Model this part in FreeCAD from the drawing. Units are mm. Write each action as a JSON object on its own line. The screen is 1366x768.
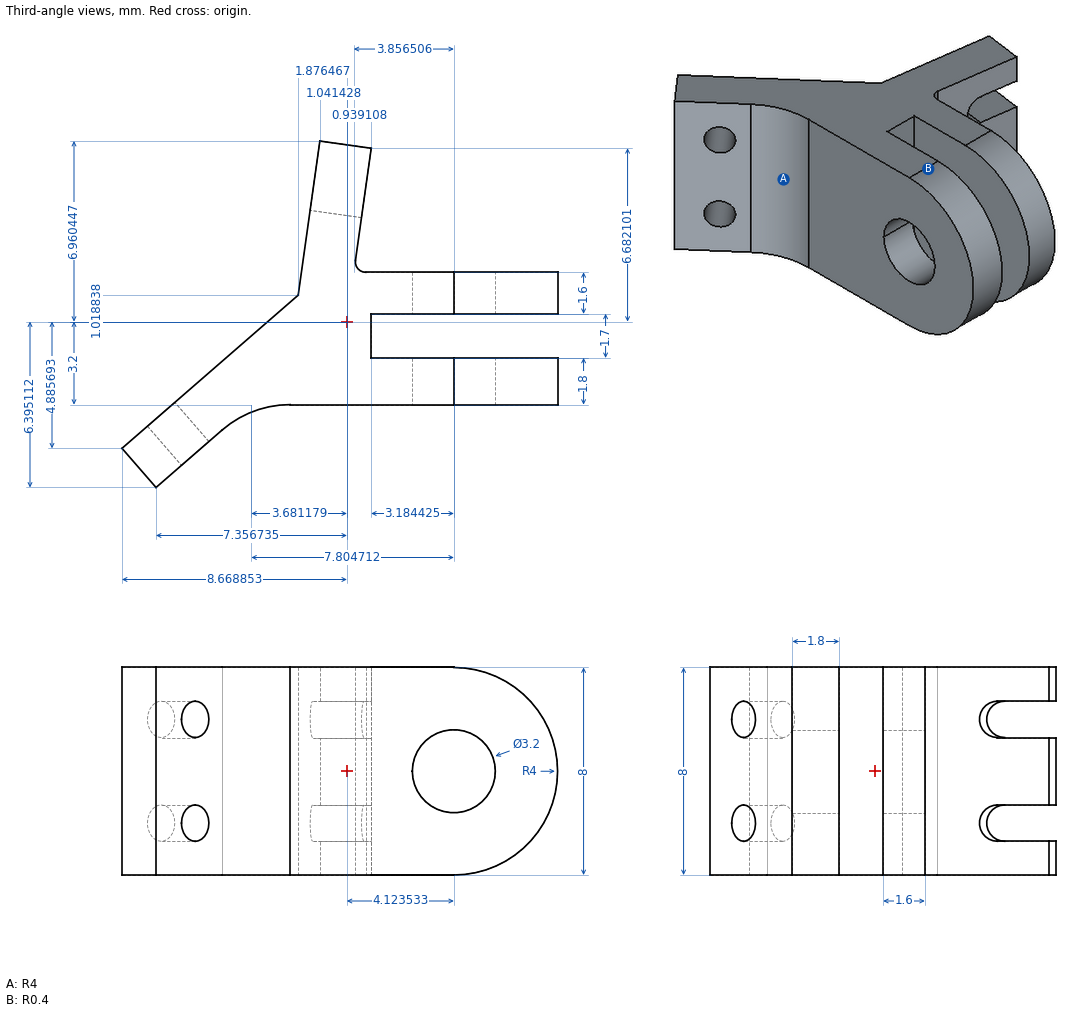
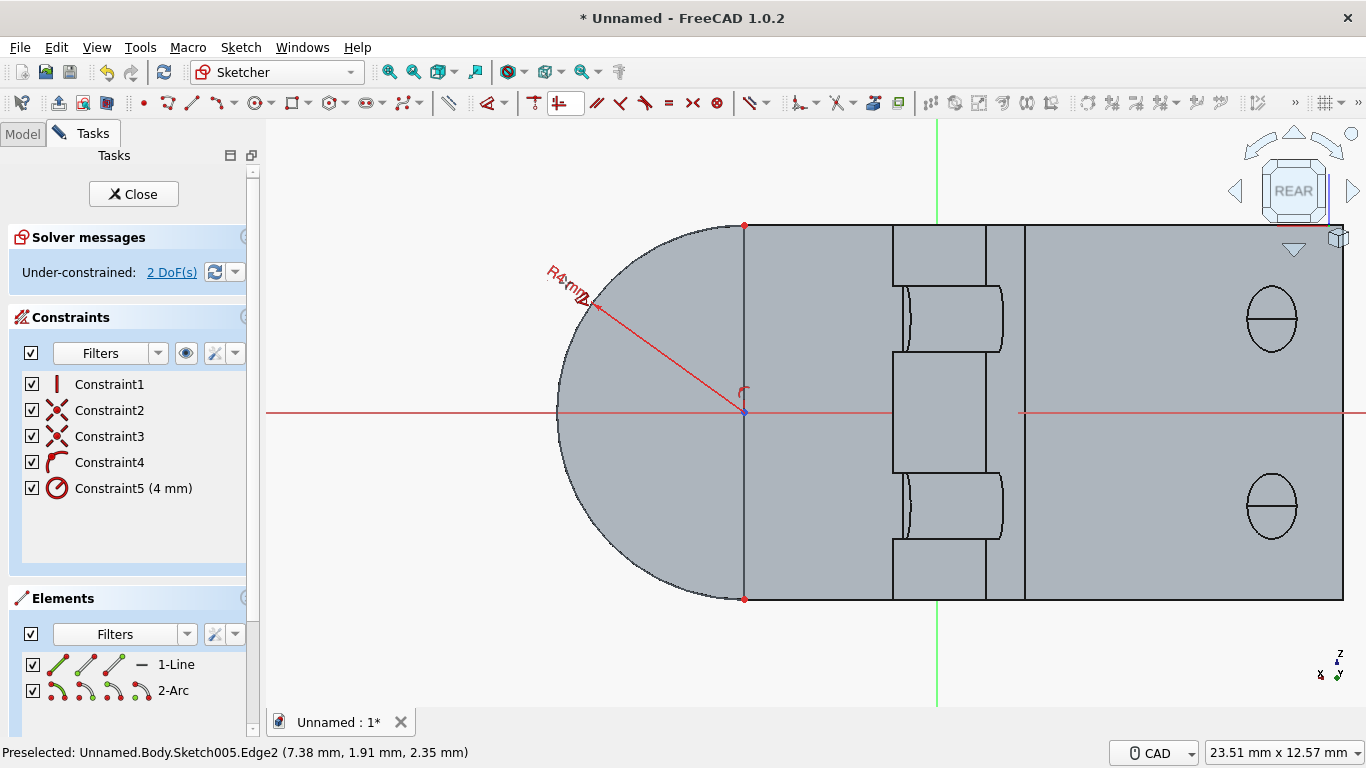
{"action": "left_click", "coordinate": [744, 600]}
{"action": "left_click", "coordinate": [840, 634]}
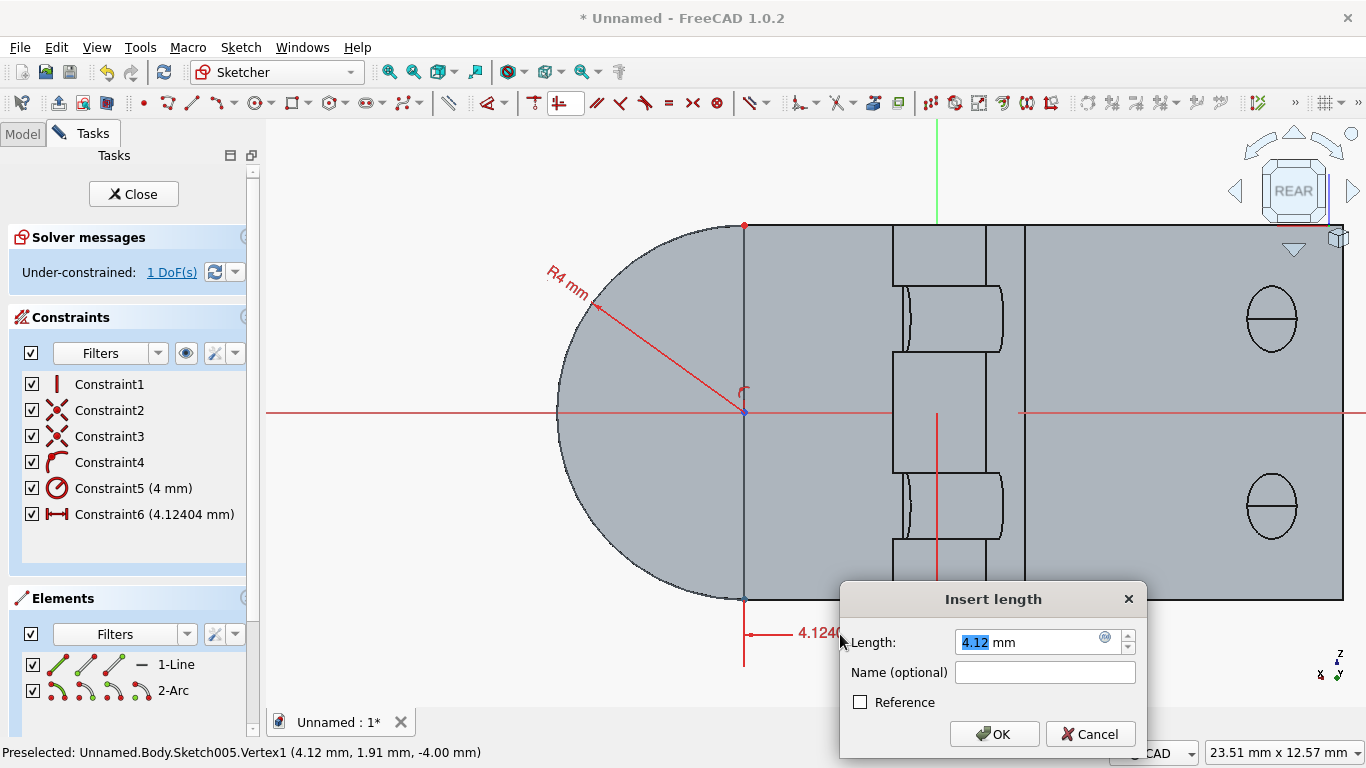
{"action": "type", "text": "4.123533"}
{"action": "key", "text": "Return"}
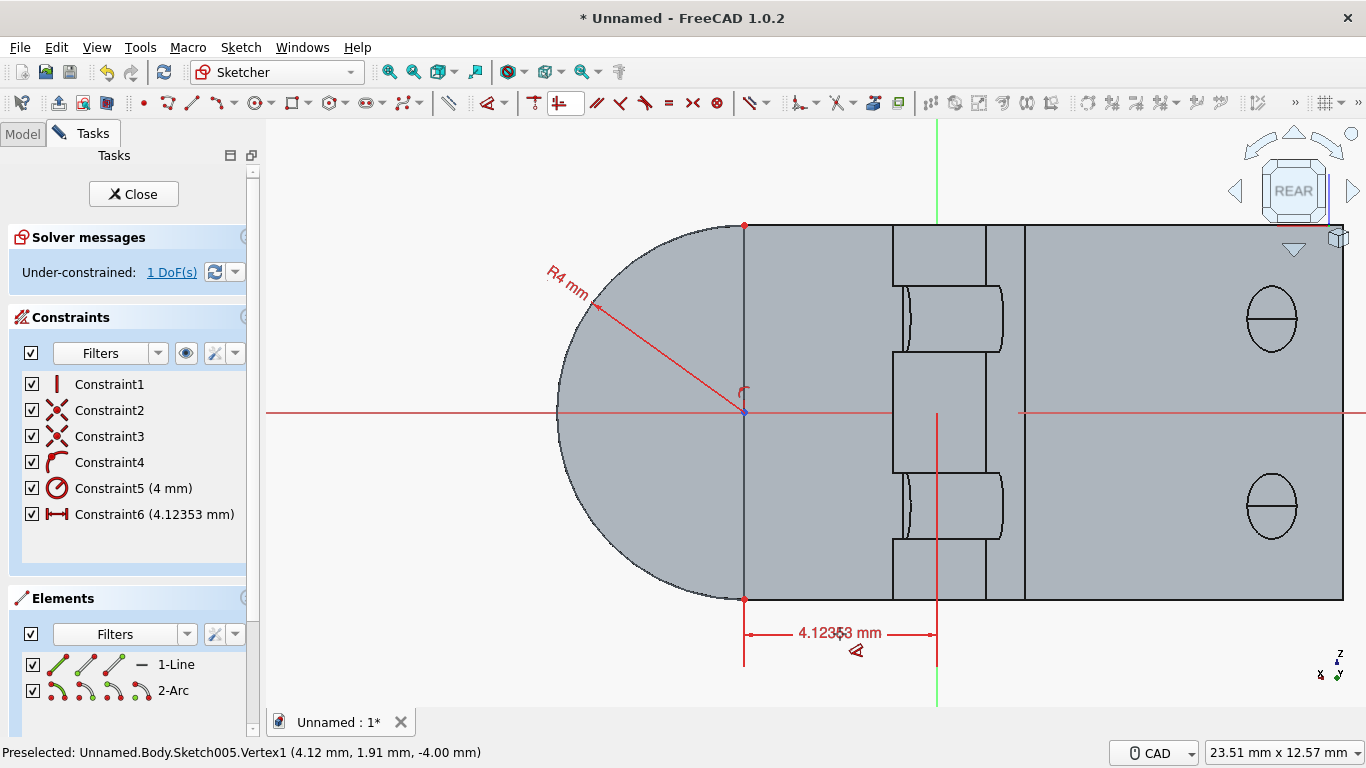
{"action": "left_click", "coordinate": [744, 413]}
{"action": "left_click", "coordinate": [841, 447]}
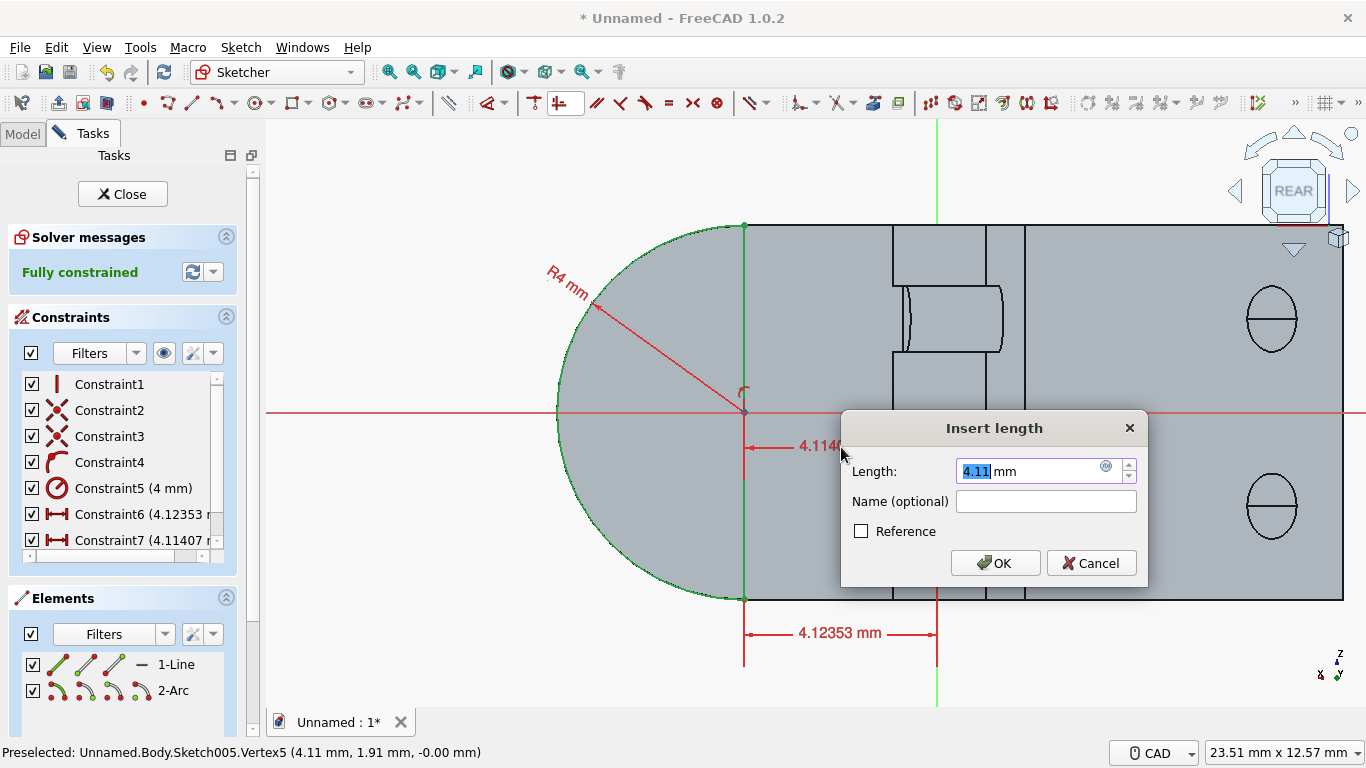
{"action": "type", "text": "4.123533"}
{"action": "key", "text": "Return"}
{"action": "key", "text": "Escape"}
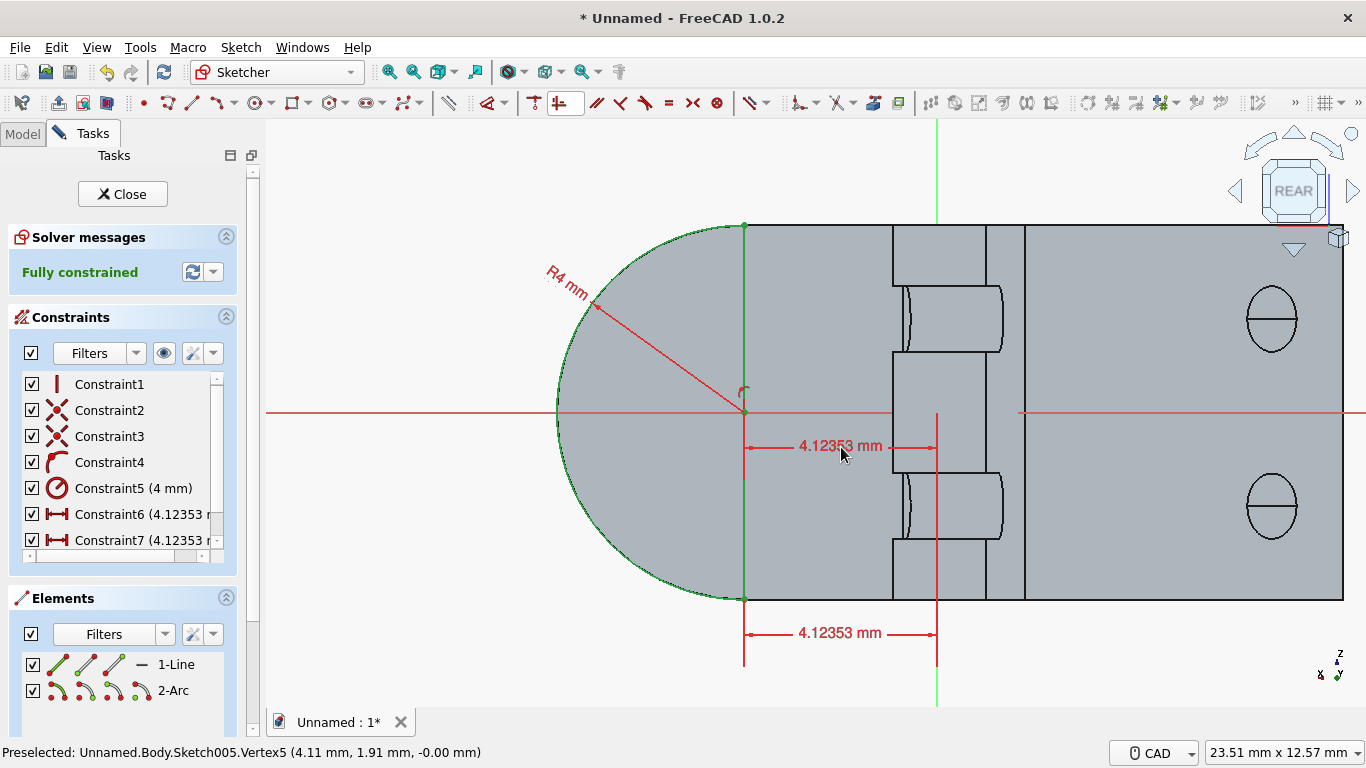
{"action": "left_click", "coordinate": [123, 194]}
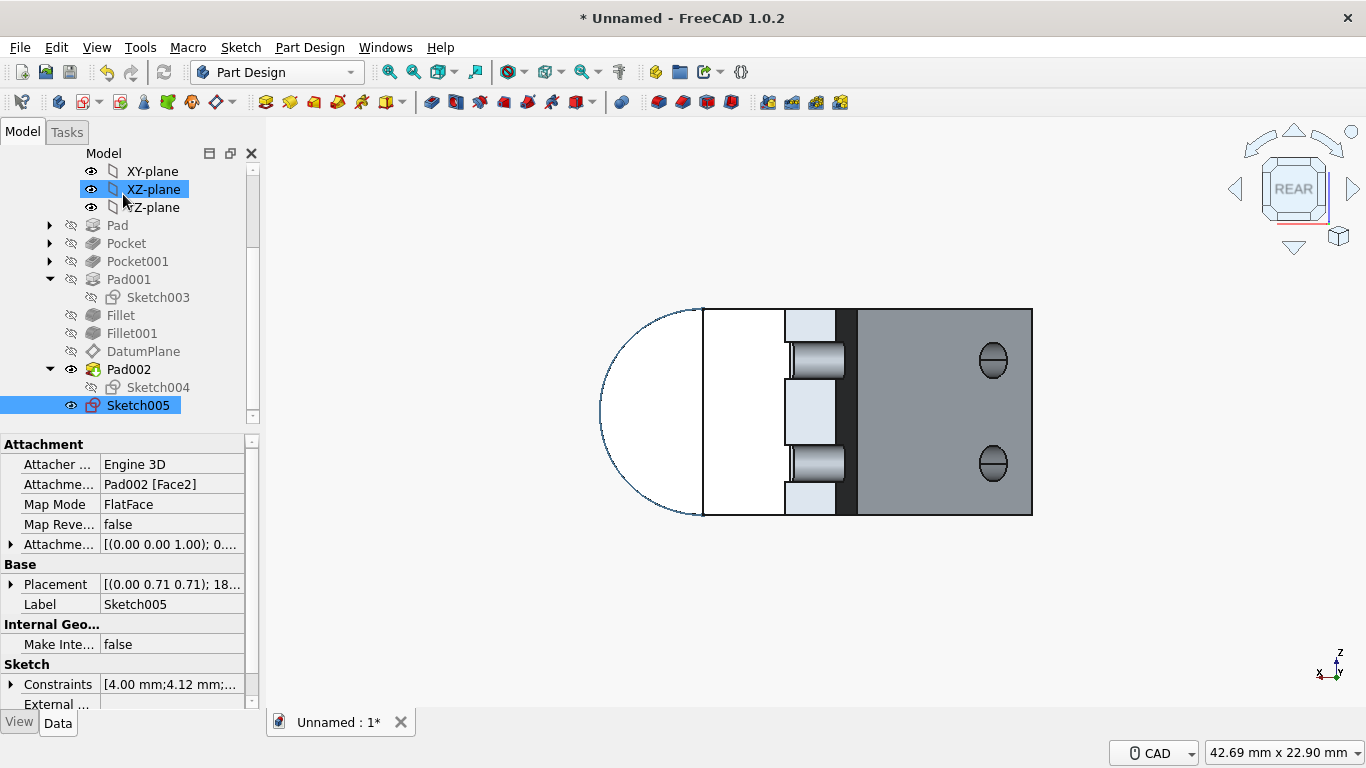
{"action": "left_click", "coordinate": [266, 102]}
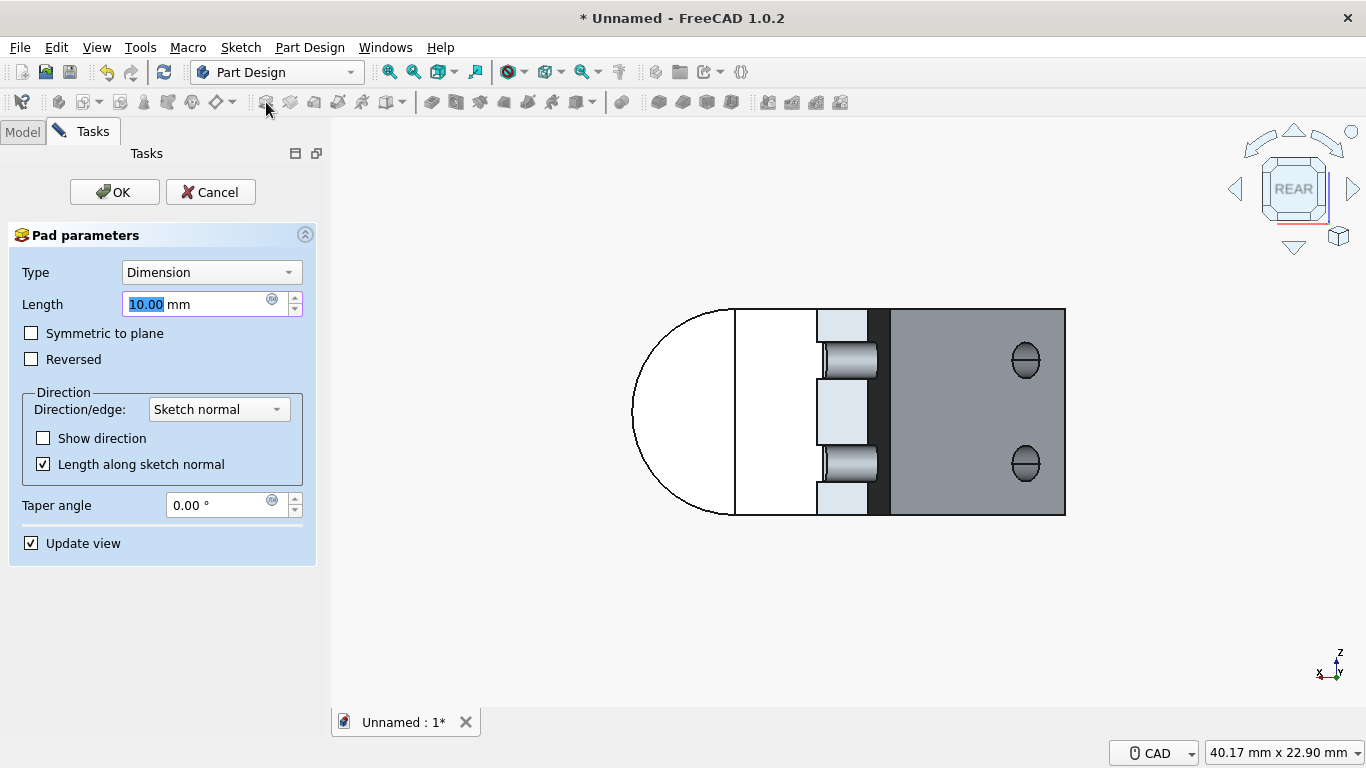
{"action": "type", "text": "1.6"}
{"action": "key", "text": "Tab"}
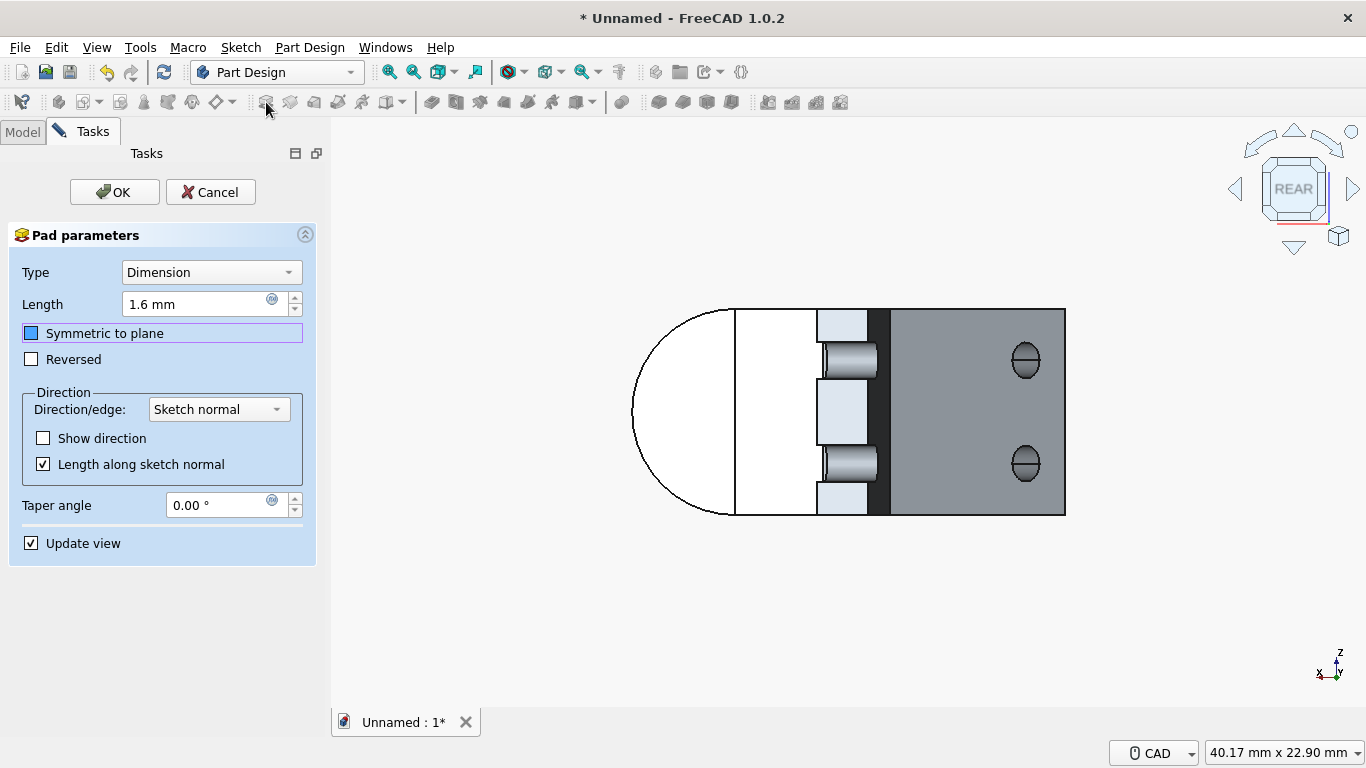
{"action": "left_click", "coordinate": [30, 359]}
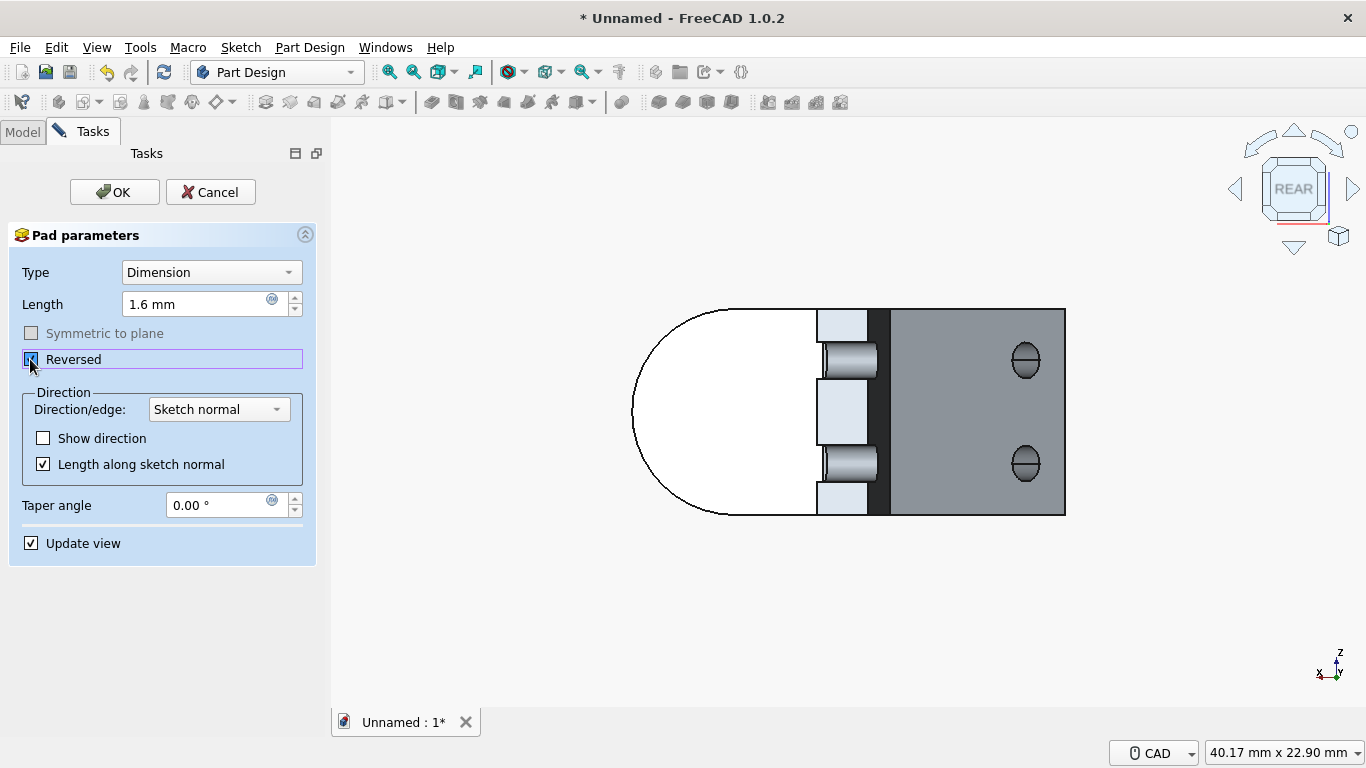
{"action": "left_click", "coordinate": [115, 192]}